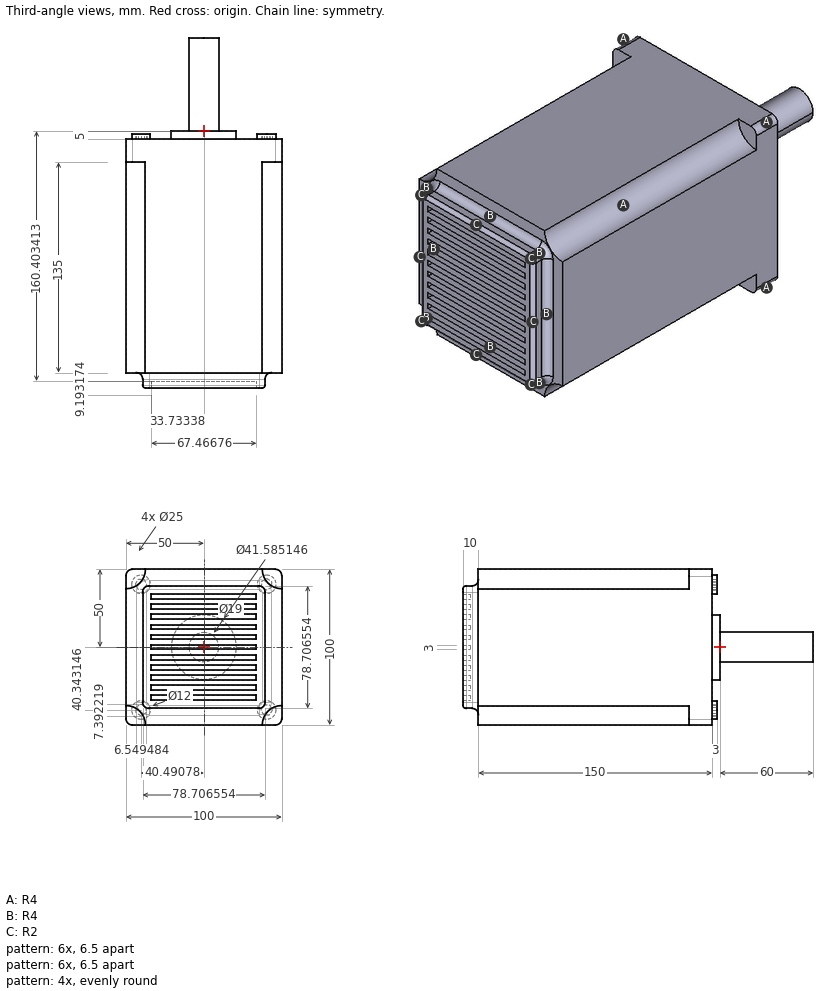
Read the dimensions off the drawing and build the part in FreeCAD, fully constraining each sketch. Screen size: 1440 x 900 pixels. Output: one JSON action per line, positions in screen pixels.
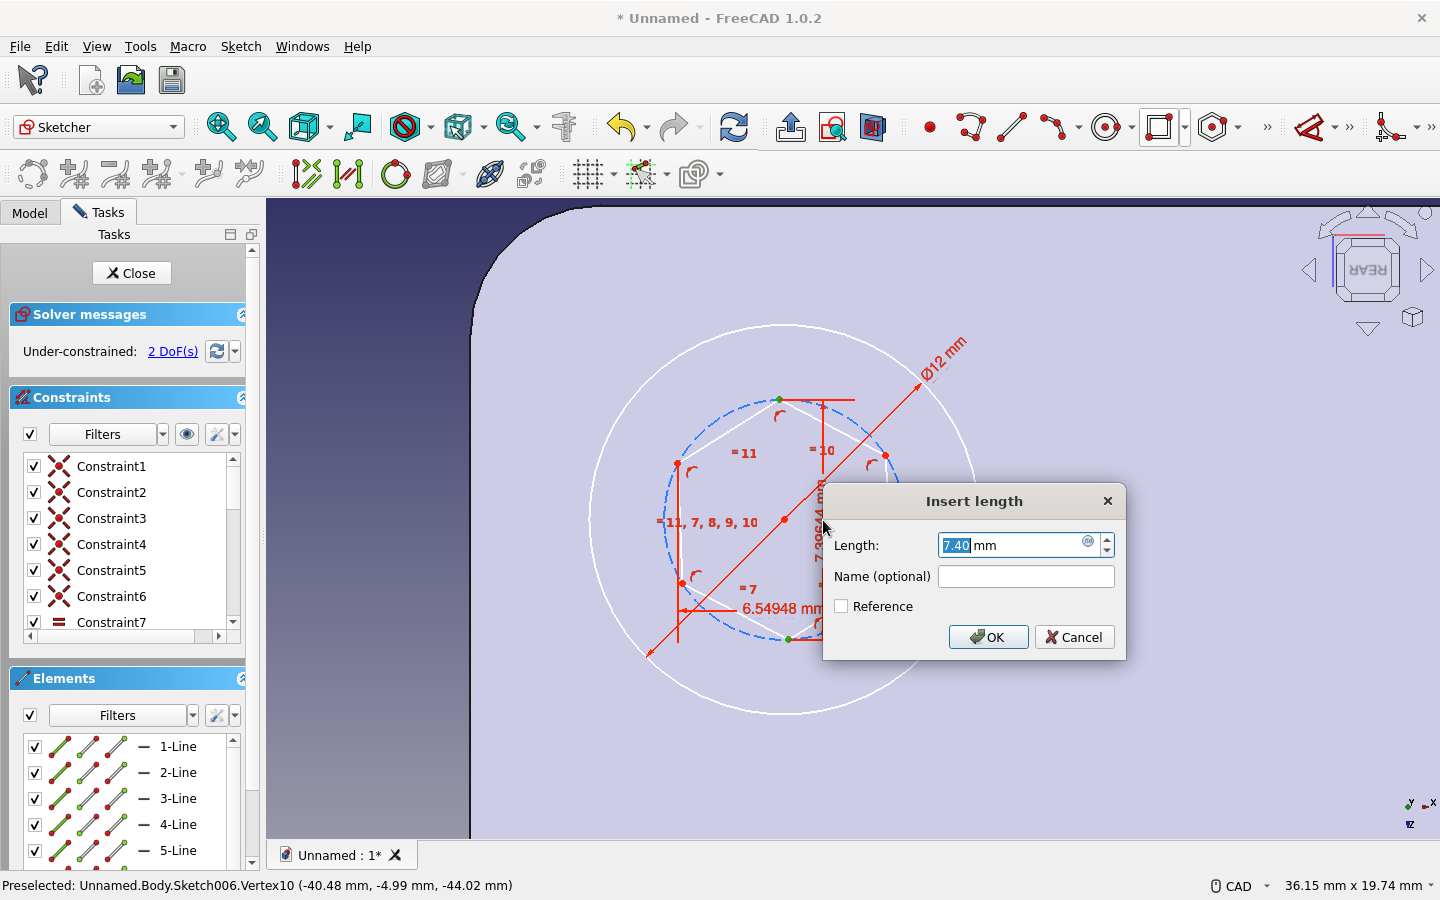
{"action": "type", "text": "7.392219"}
{"action": "key", "text": "Return"}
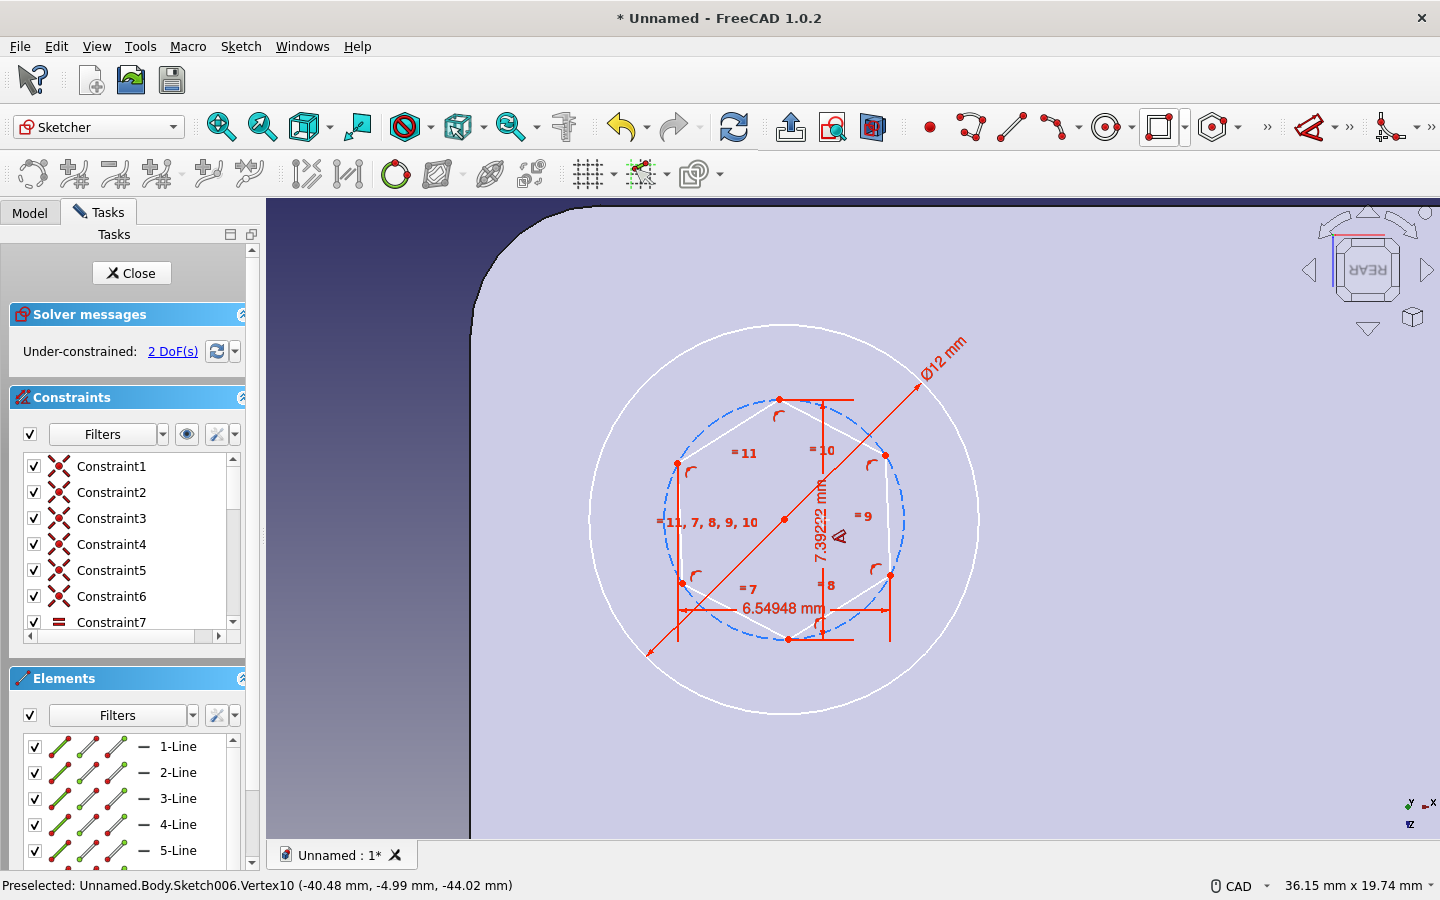
{"action": "left_click", "coordinate": [779, 400]}
{"action": "left_click", "coordinate": [1027, 366]}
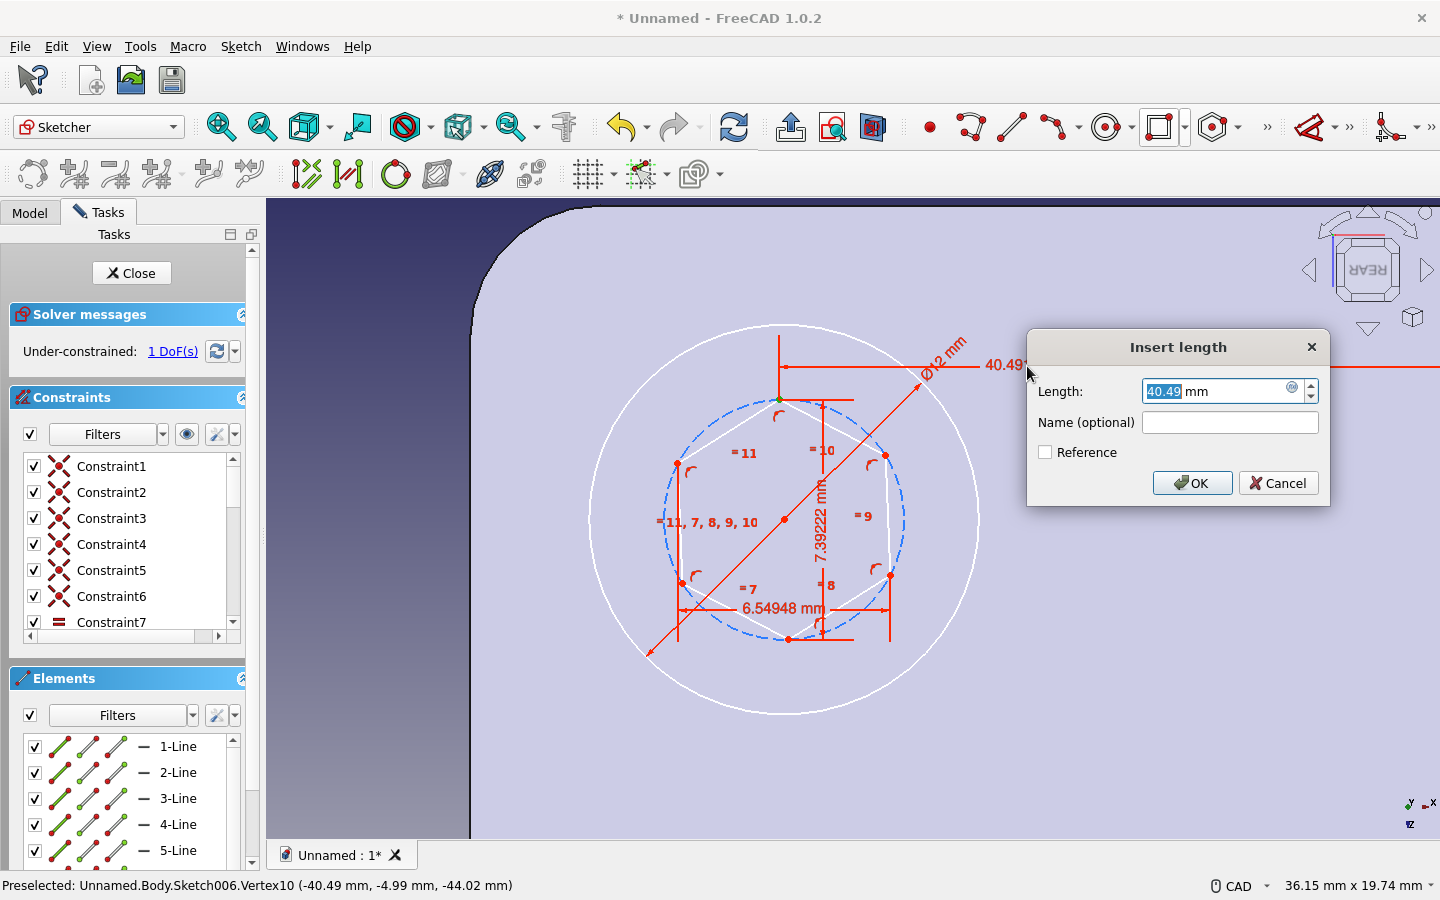
{"action": "type", "text": "40.49078"}
{"action": "key", "text": "Return"}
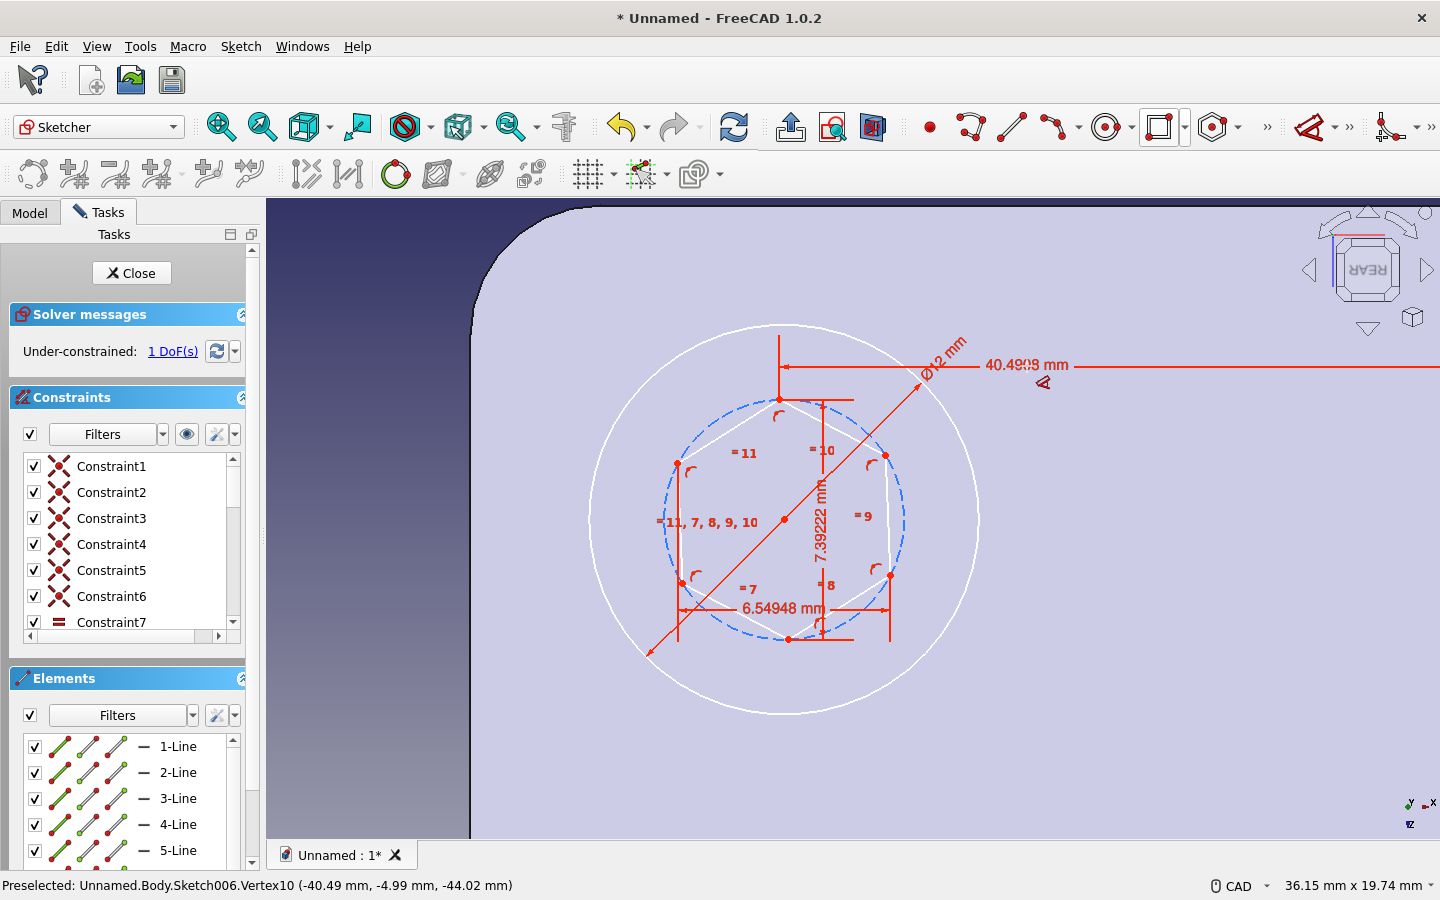
{"action": "left_click", "coordinate": [784, 520]}
{"action": "left_click", "coordinate": [750, 665]}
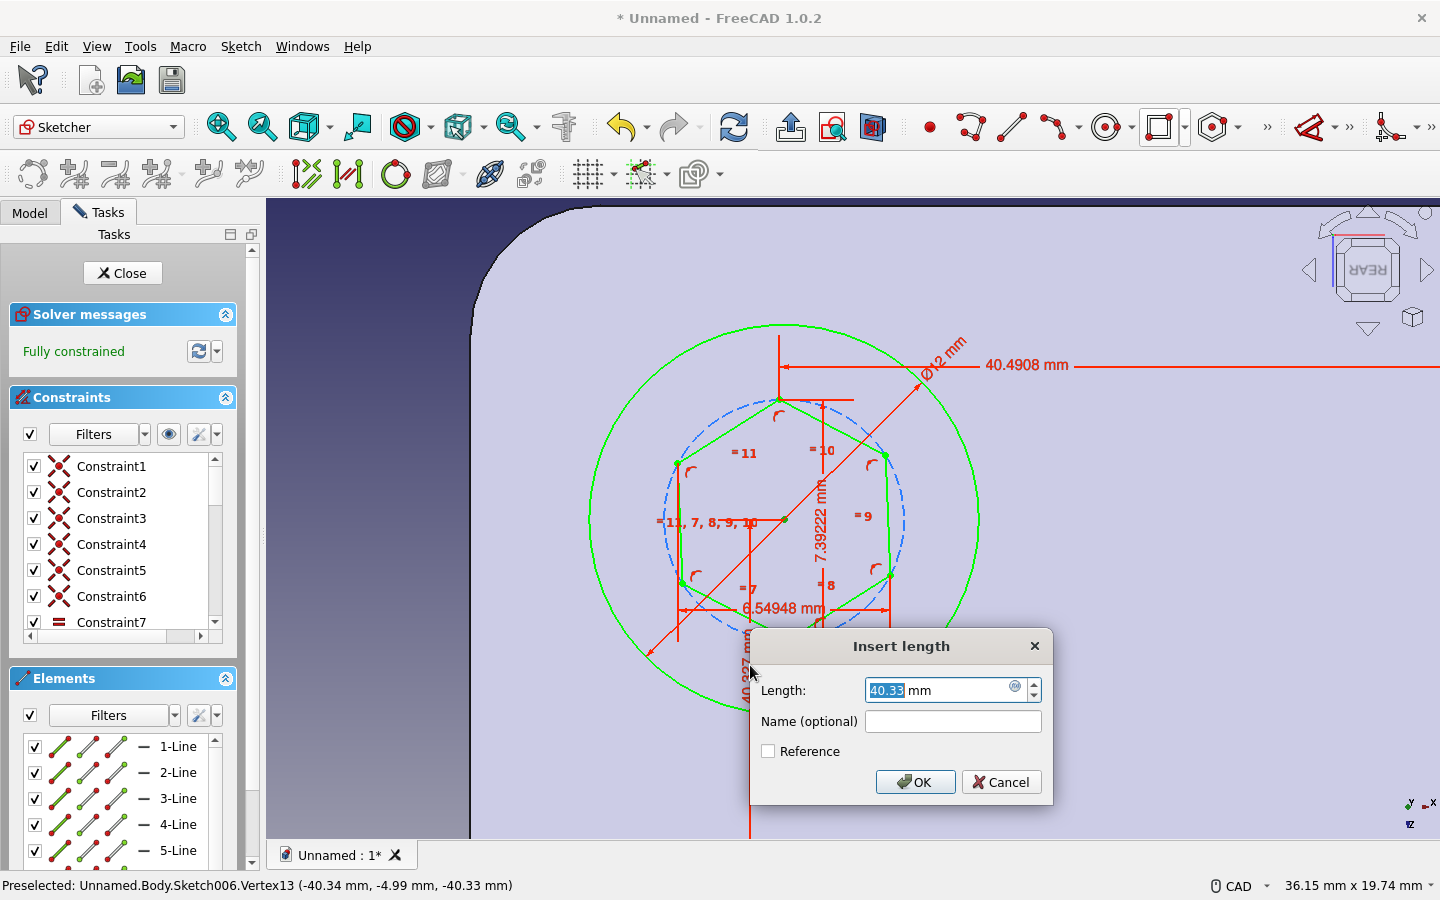
{"action": "type", "text": "40.343146"}
{"action": "key", "text": "Return"}
{"action": "key", "text": "Escape"}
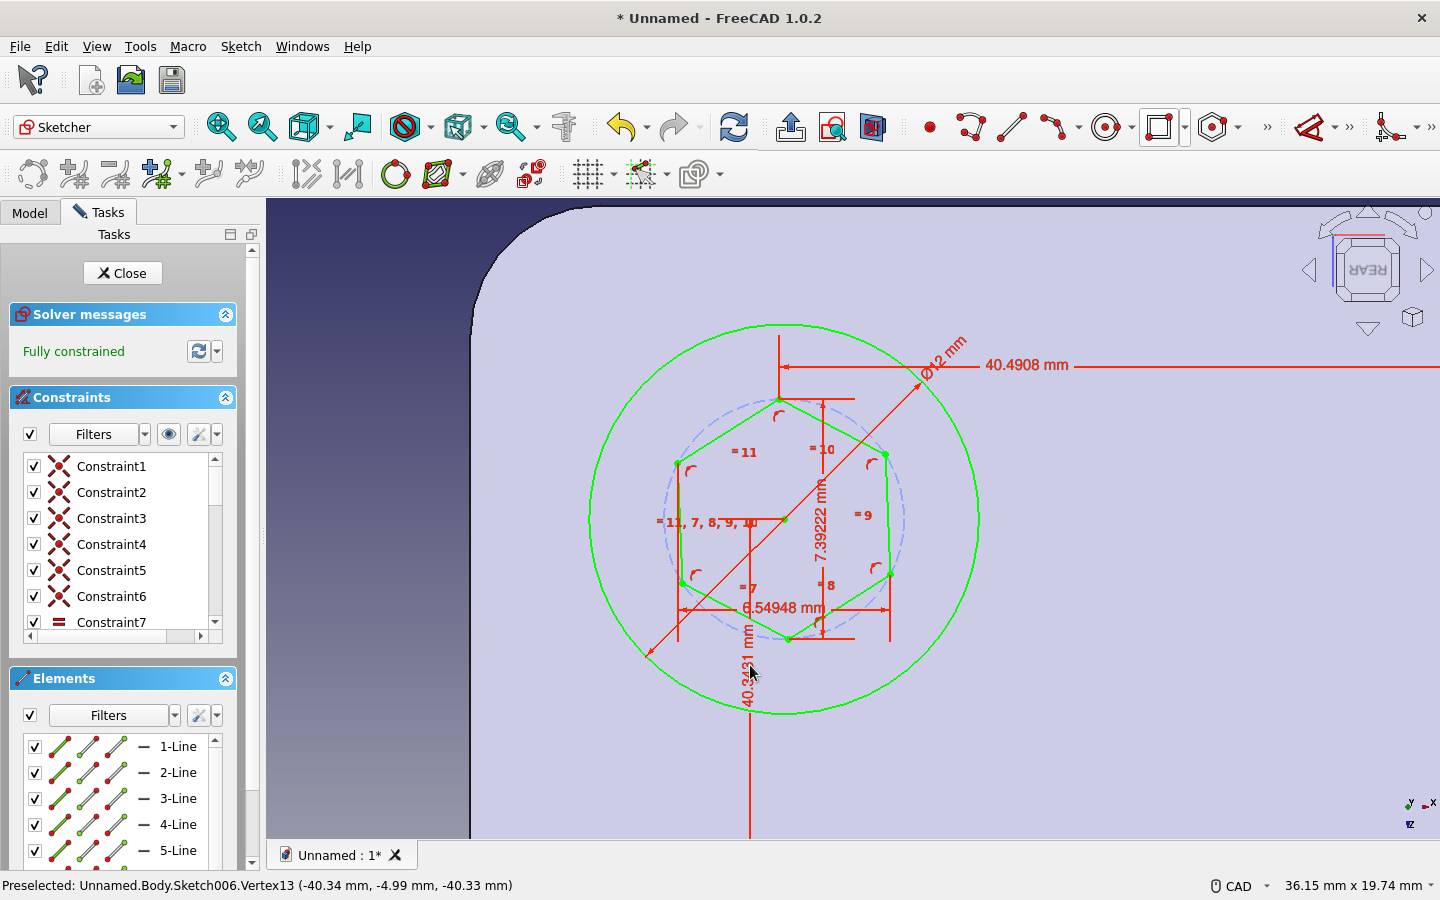
{"action": "left_click", "coordinate": [123, 273]}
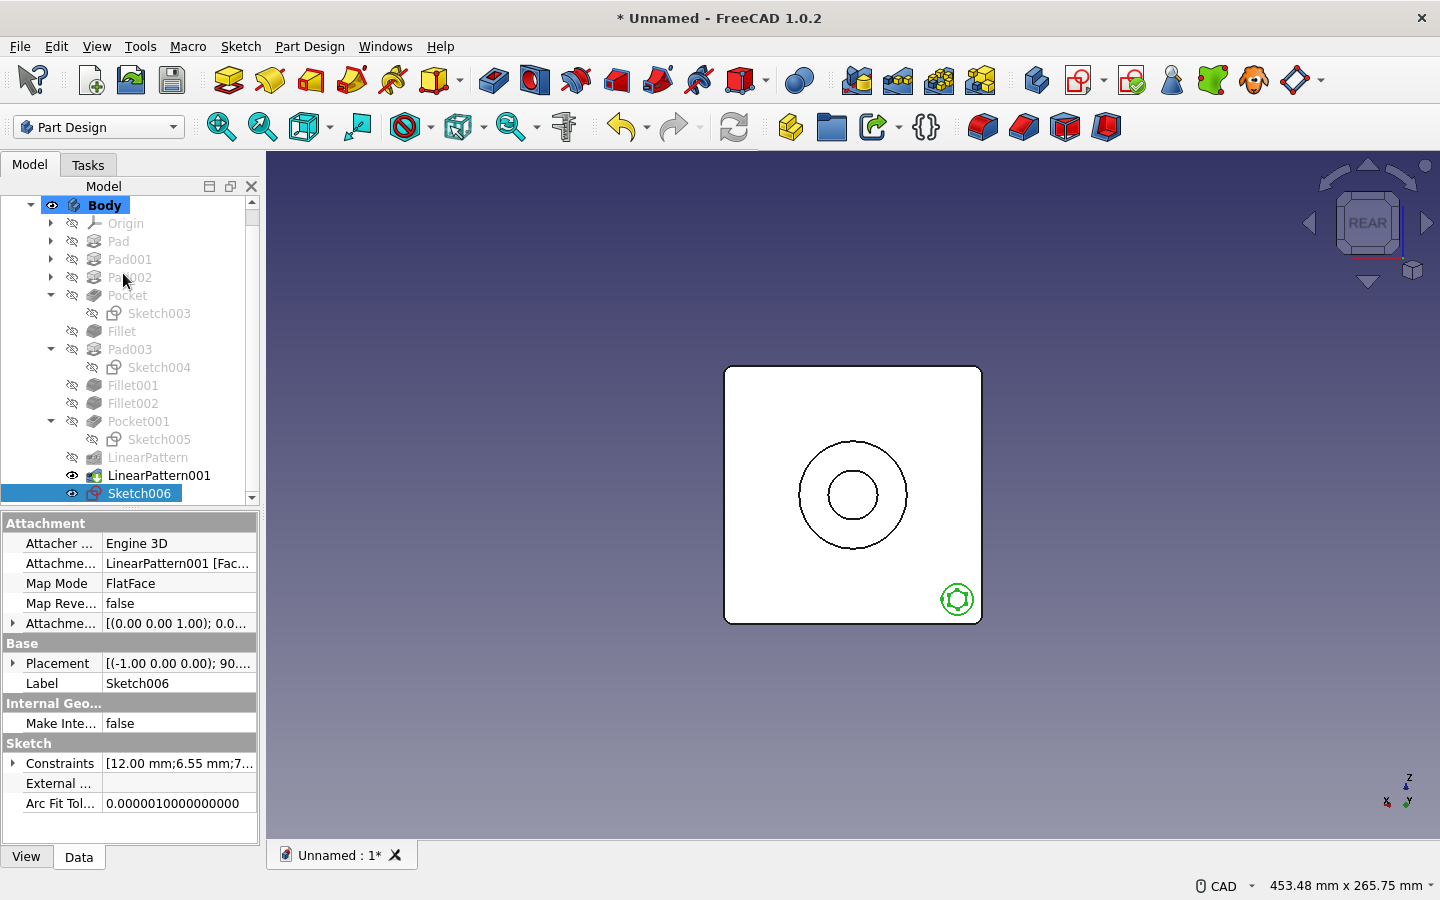
{"action": "left_click", "coordinate": [229, 80]}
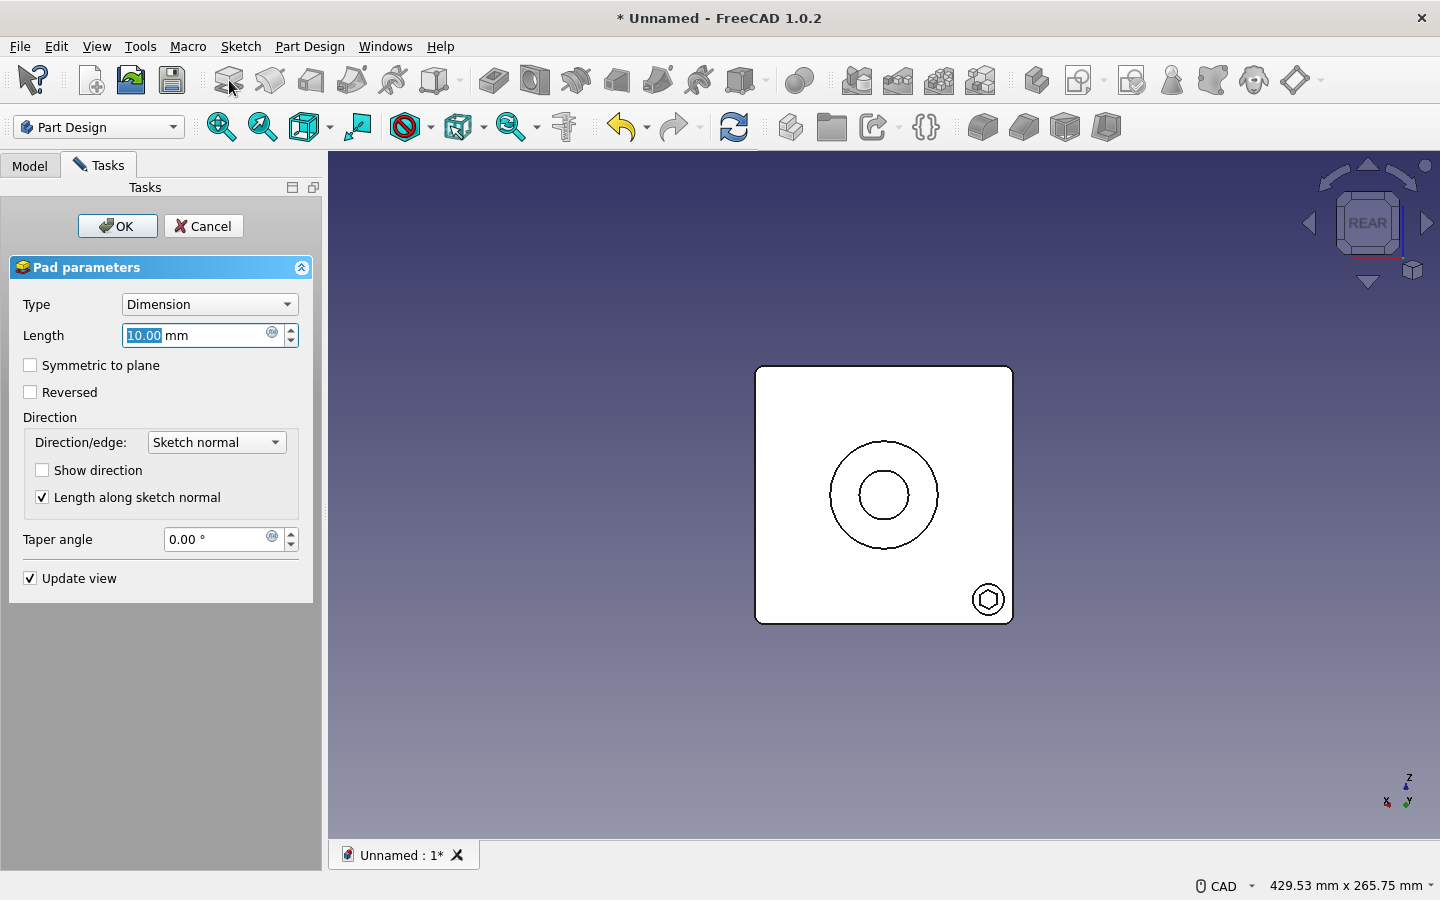
{"action": "type", "text": "3"}
{"action": "key", "text": "Tab"}